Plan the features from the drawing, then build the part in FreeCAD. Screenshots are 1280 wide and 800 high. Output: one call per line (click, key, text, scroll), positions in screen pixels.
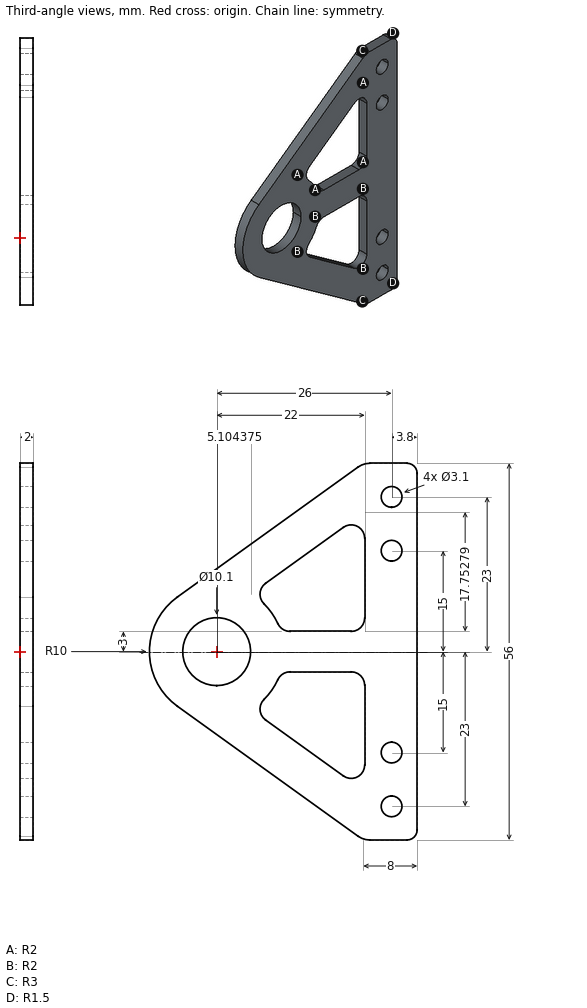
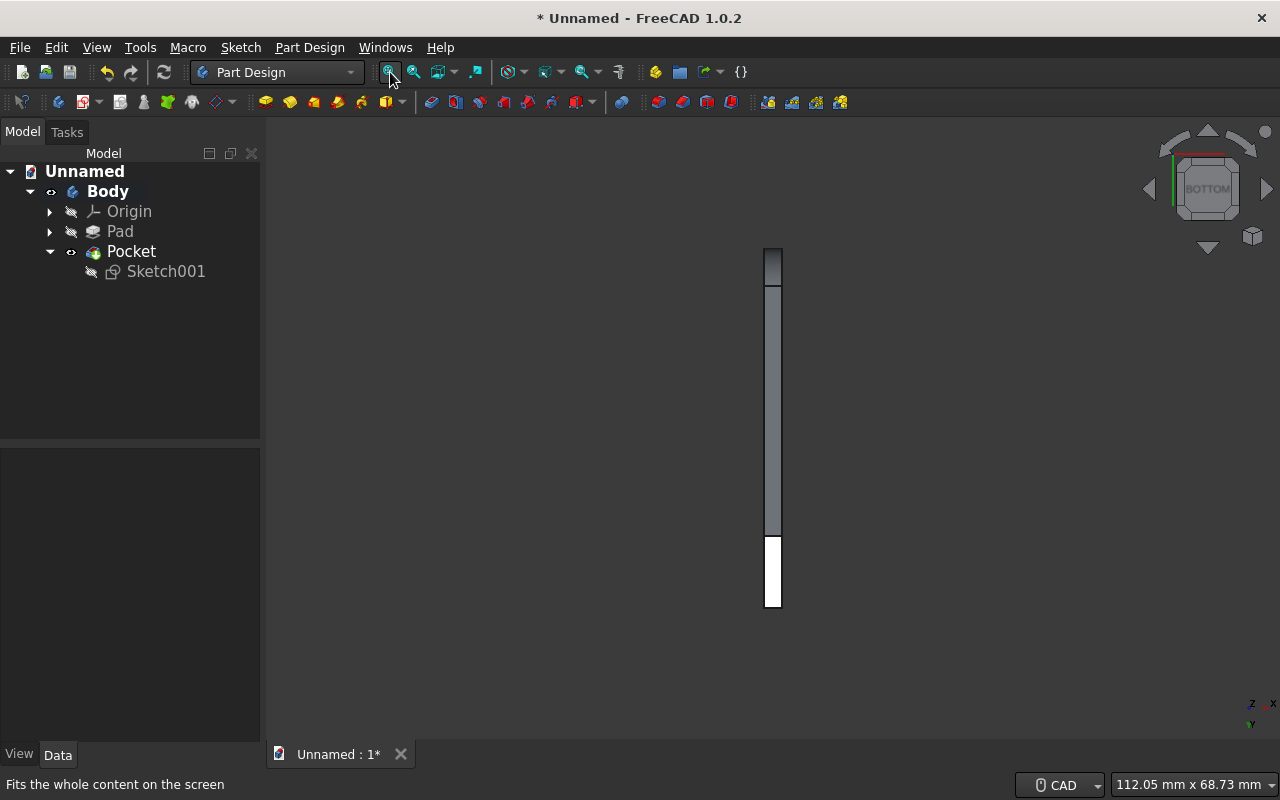
scroll(773, 537, up, 4)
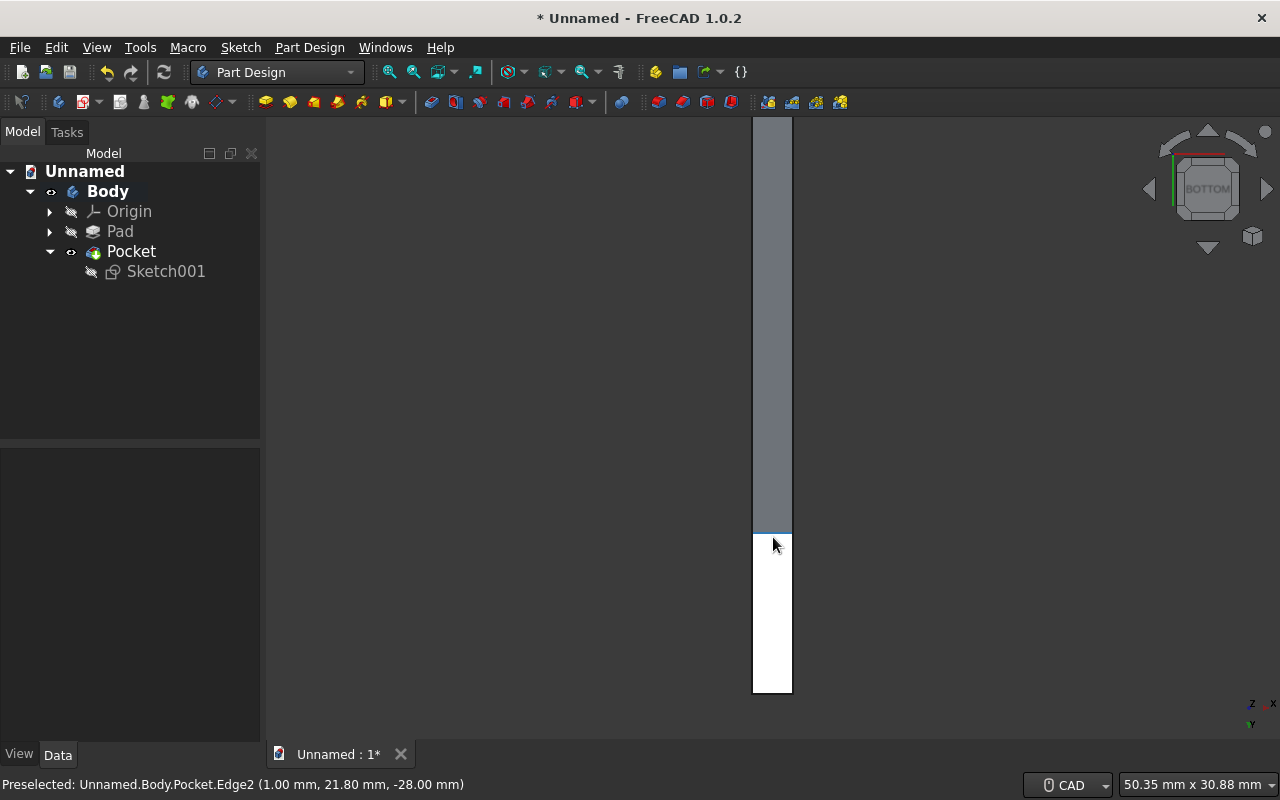
key(v)
key(f)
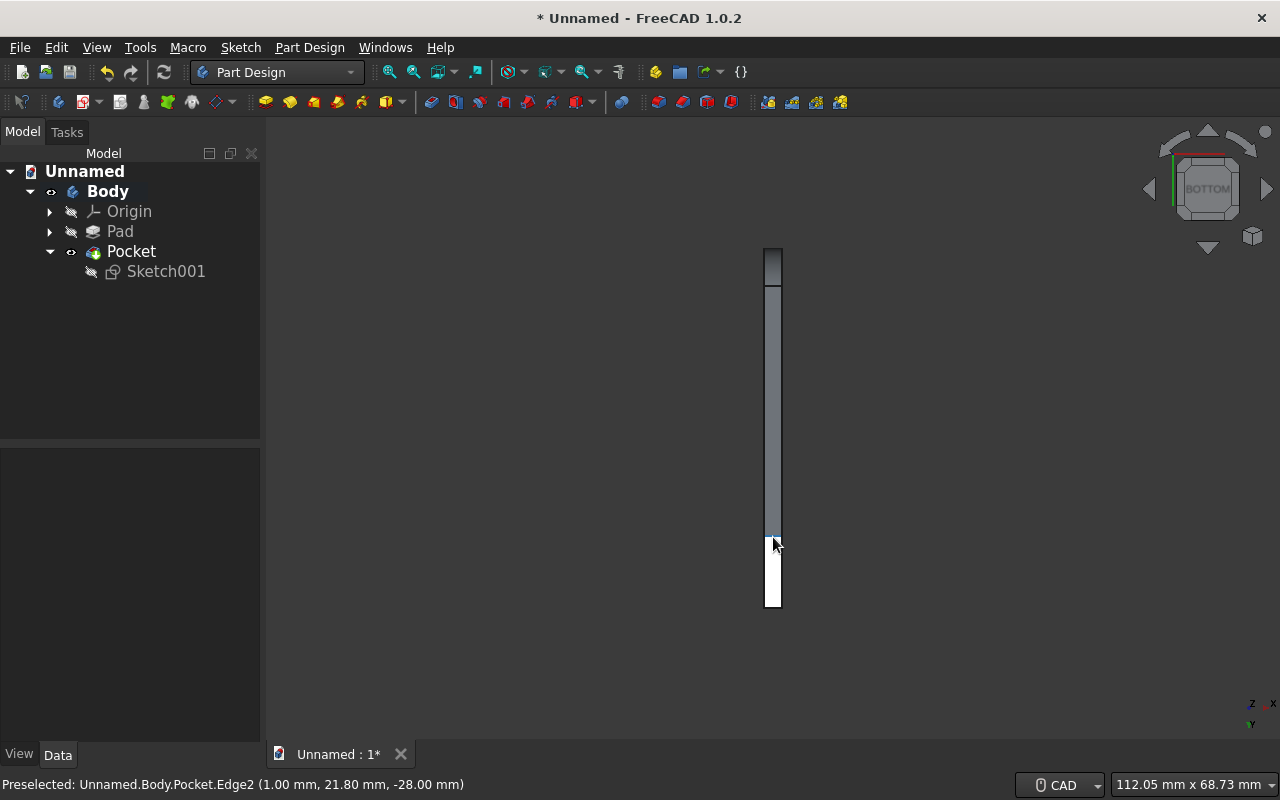
key(4)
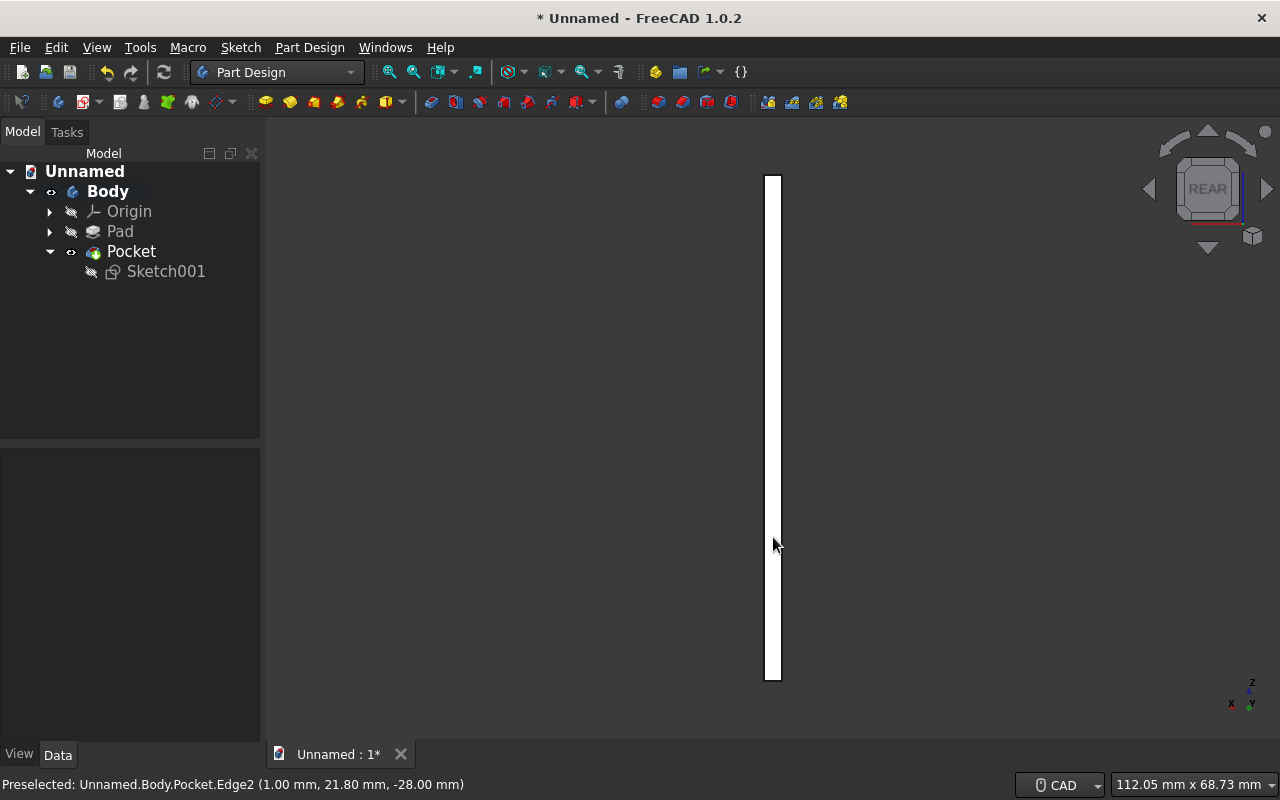
scroll(773, 400, up, 4)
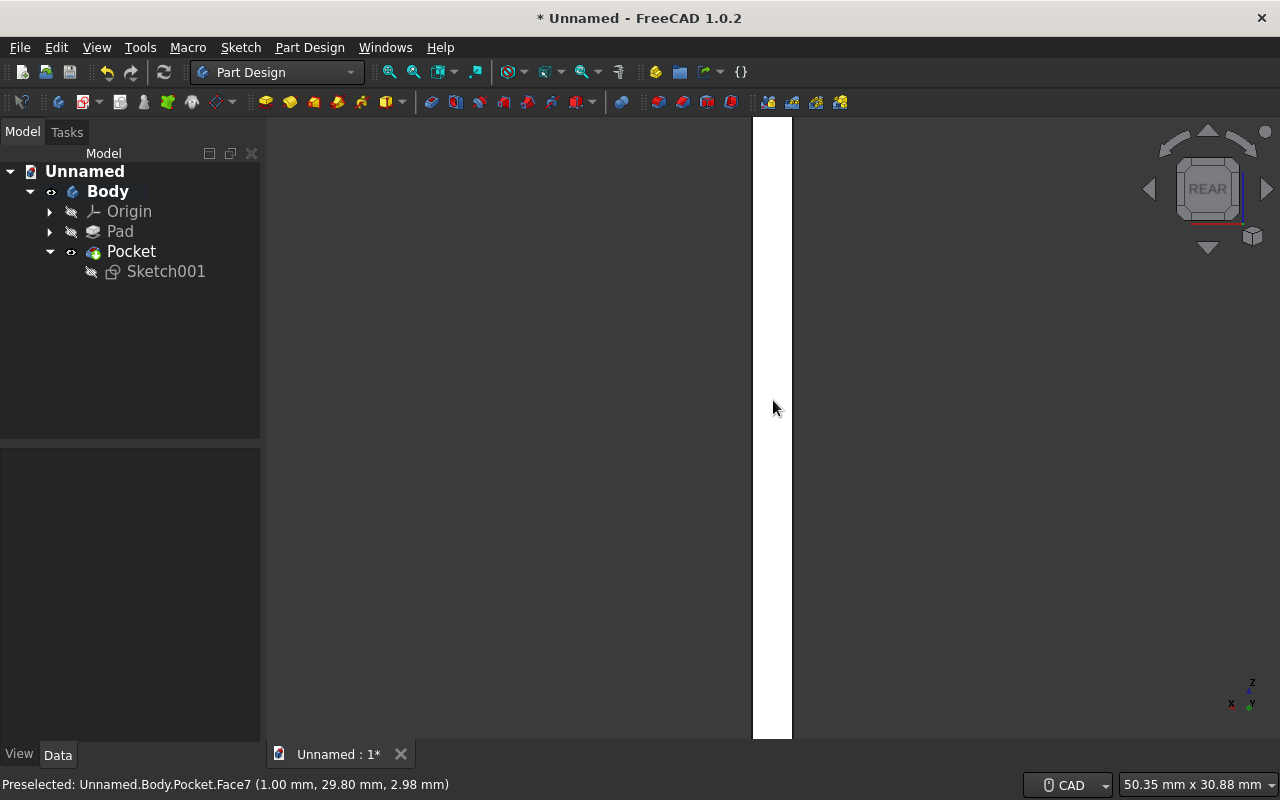
click(390, 72)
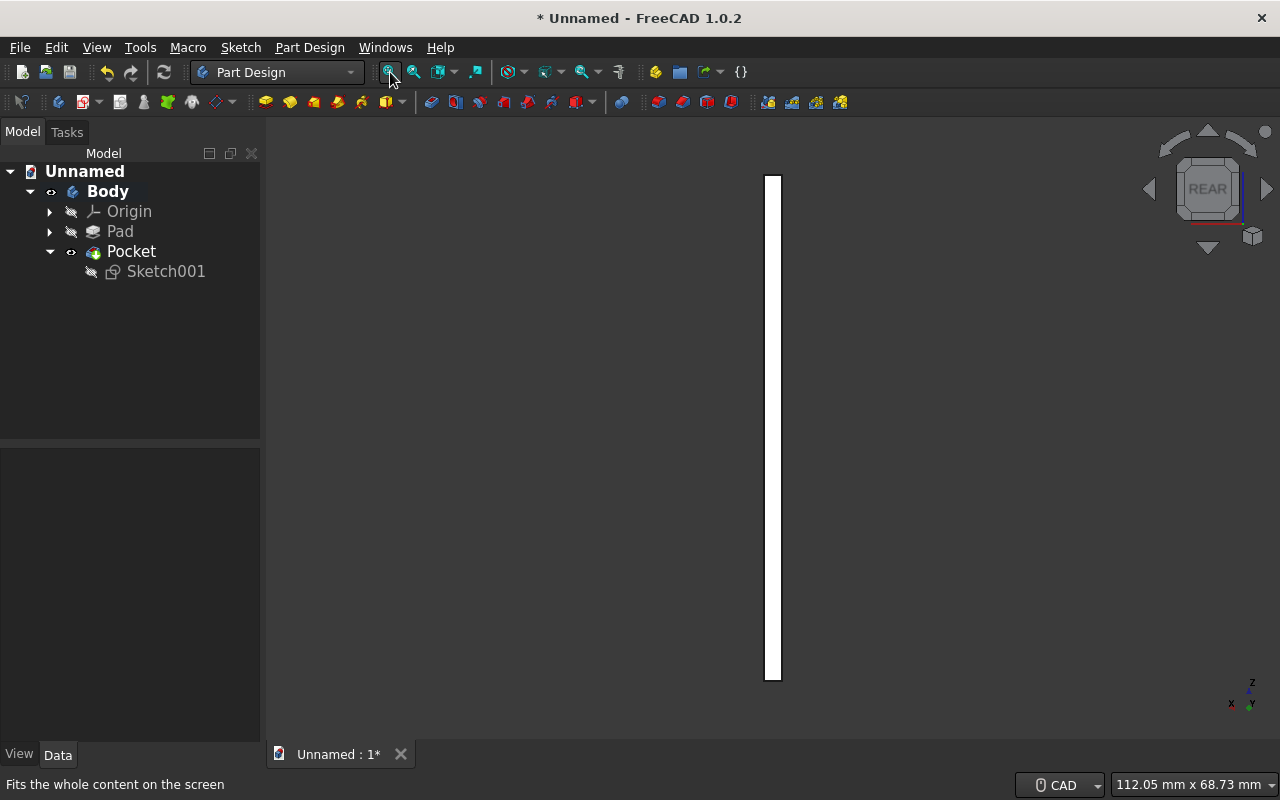
key(6)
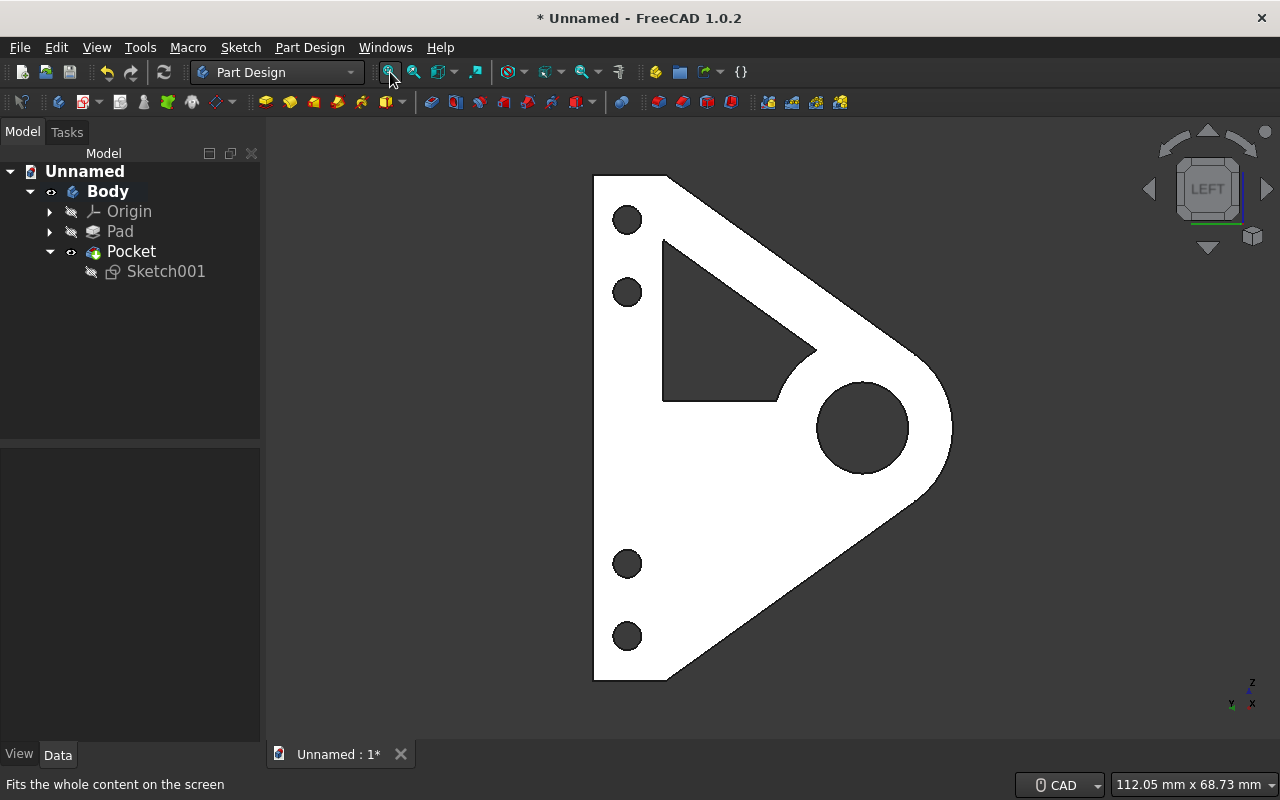
scroll(663, 400, up, 4)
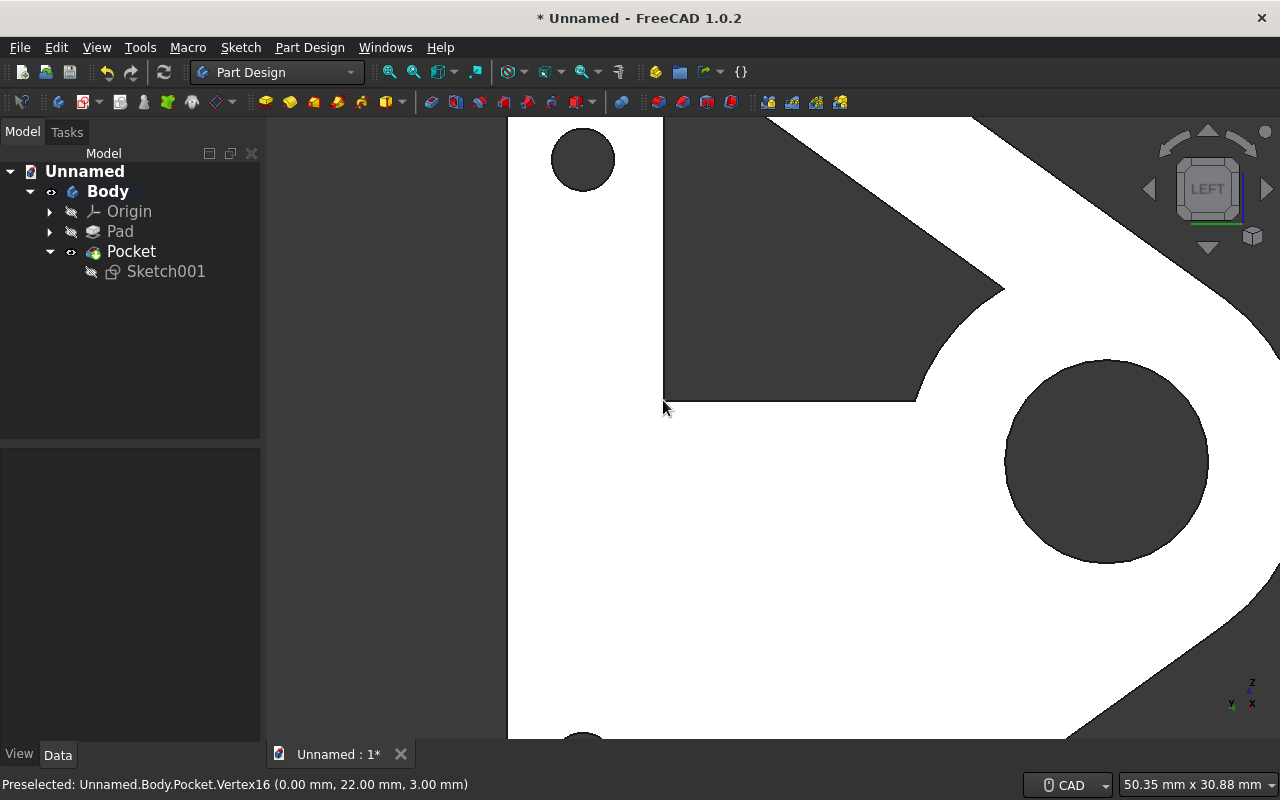
click(390, 72)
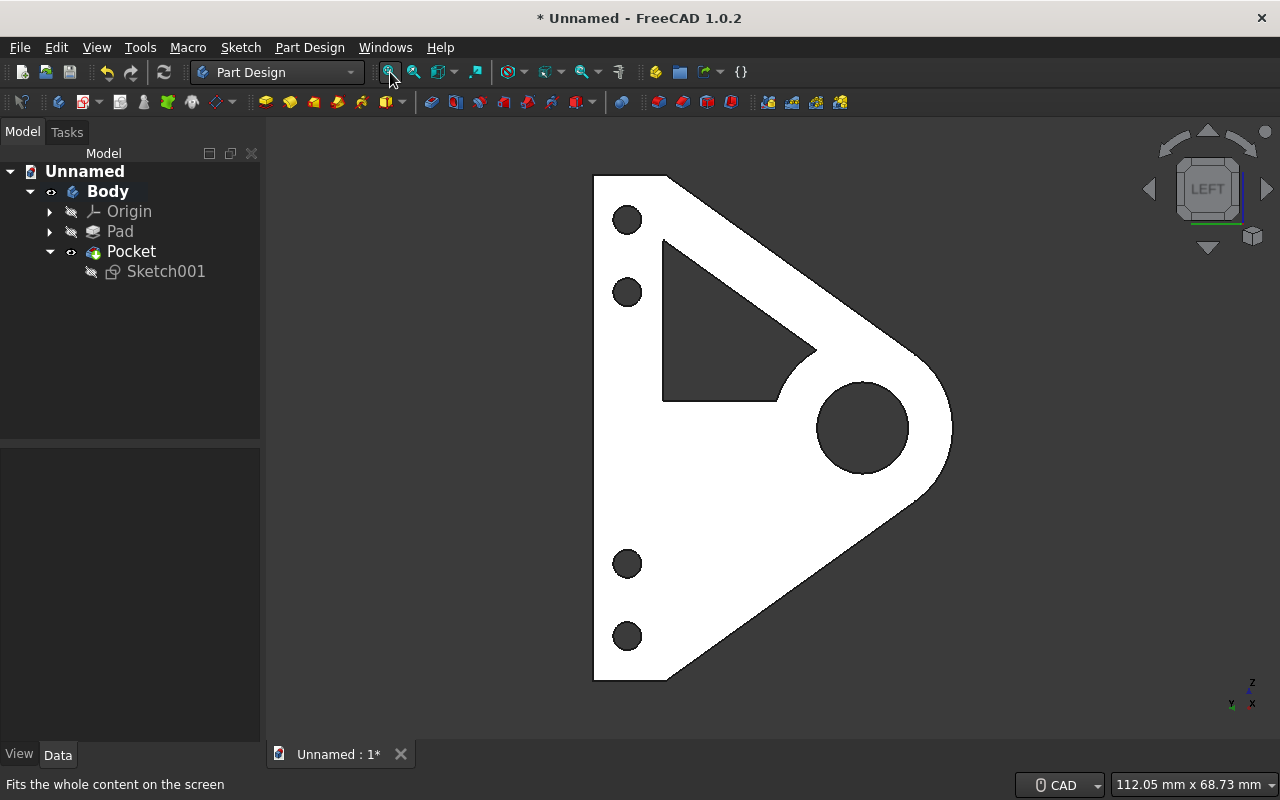
key(v)
key(3)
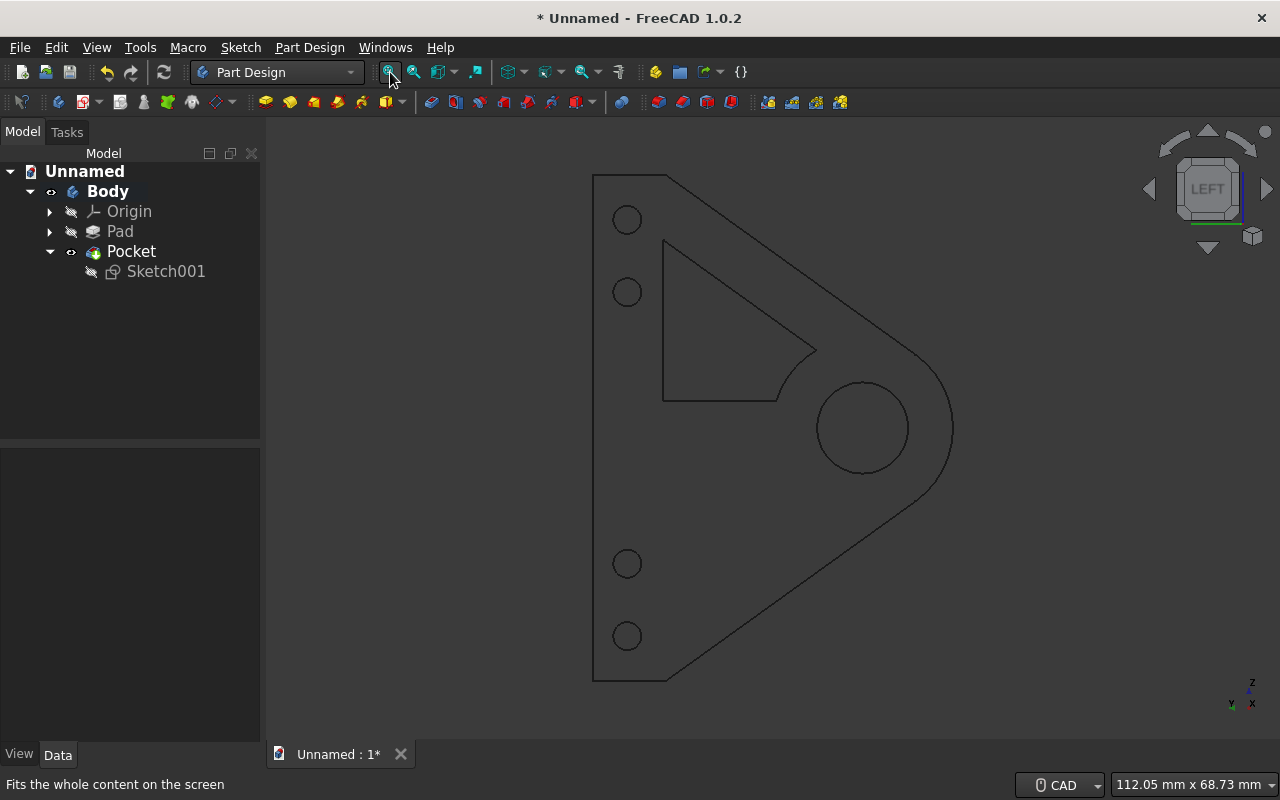
key(0)